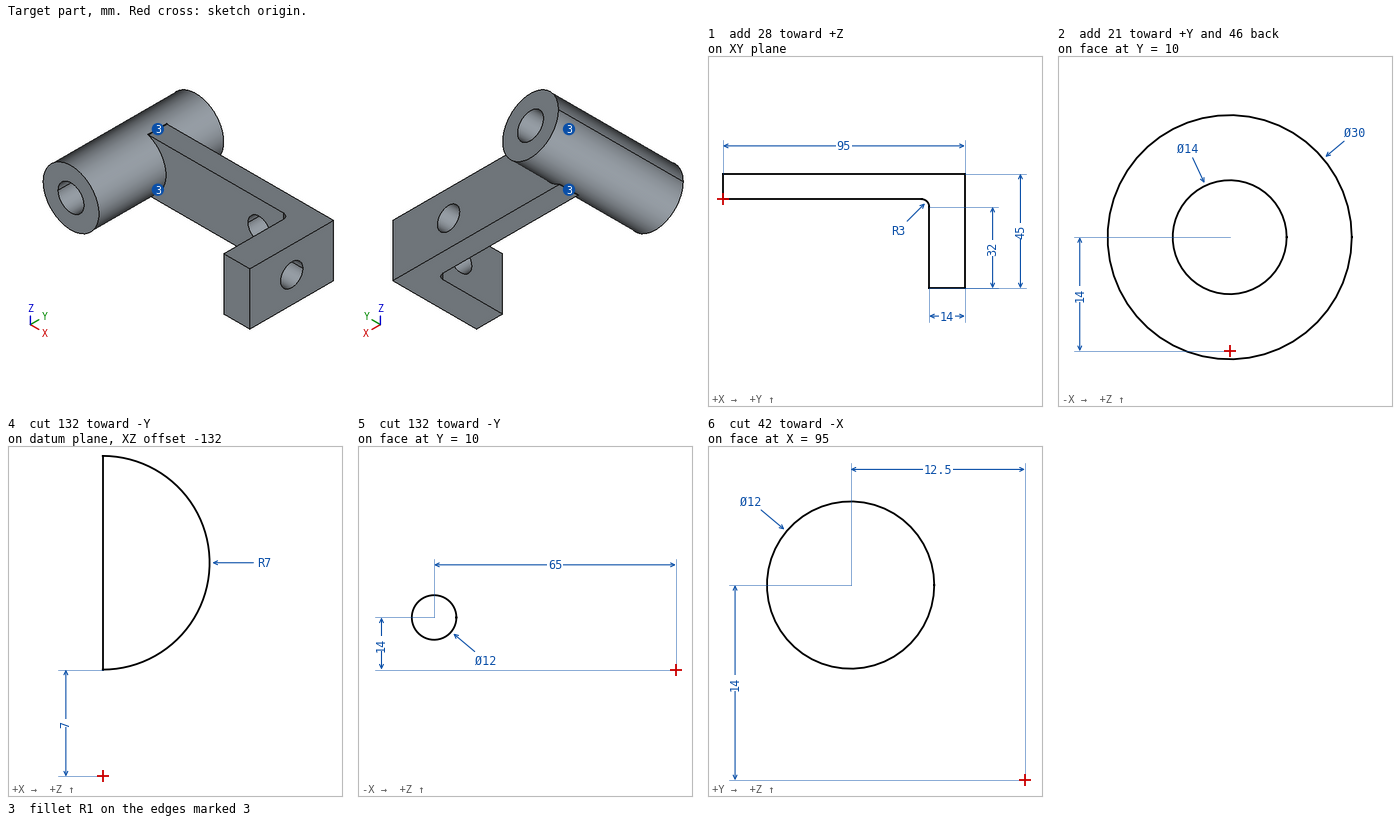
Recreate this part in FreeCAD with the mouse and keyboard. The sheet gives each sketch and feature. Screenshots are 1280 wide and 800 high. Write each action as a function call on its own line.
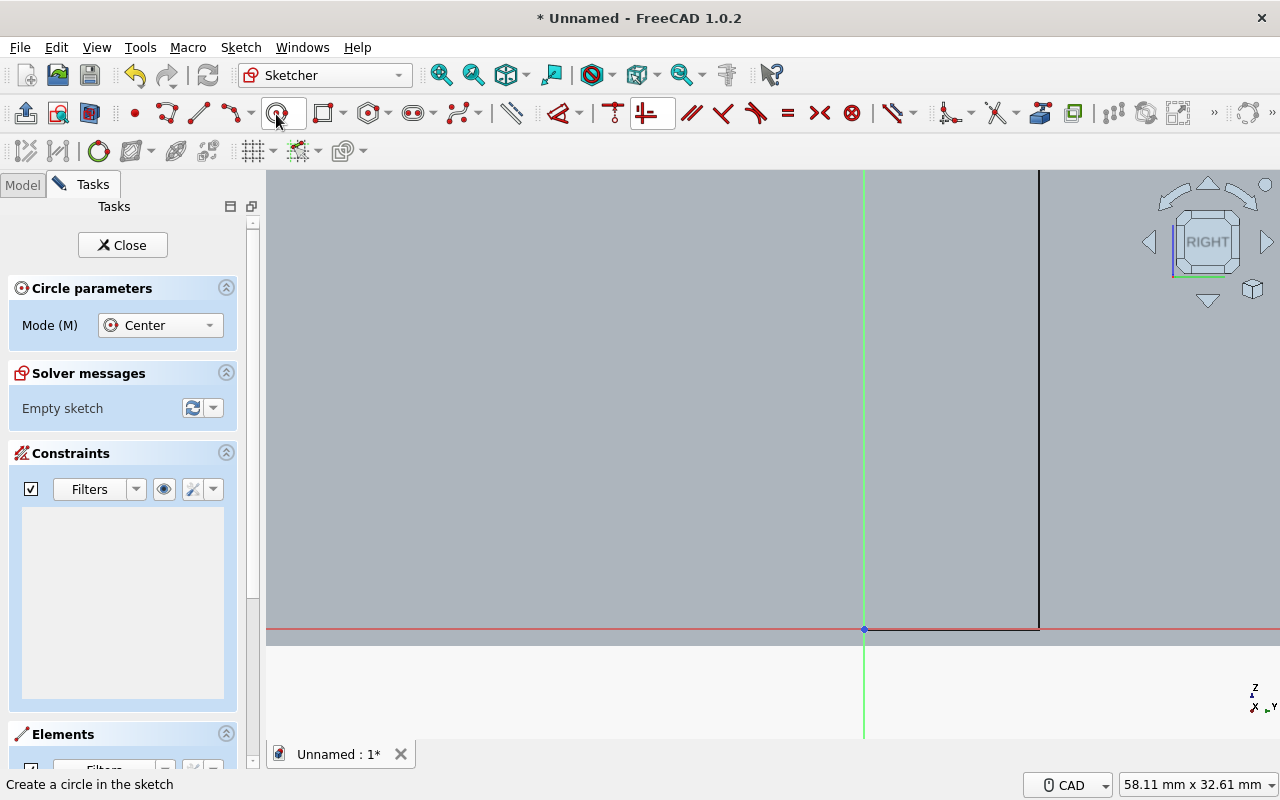
click(646, 385)
move(720, 311)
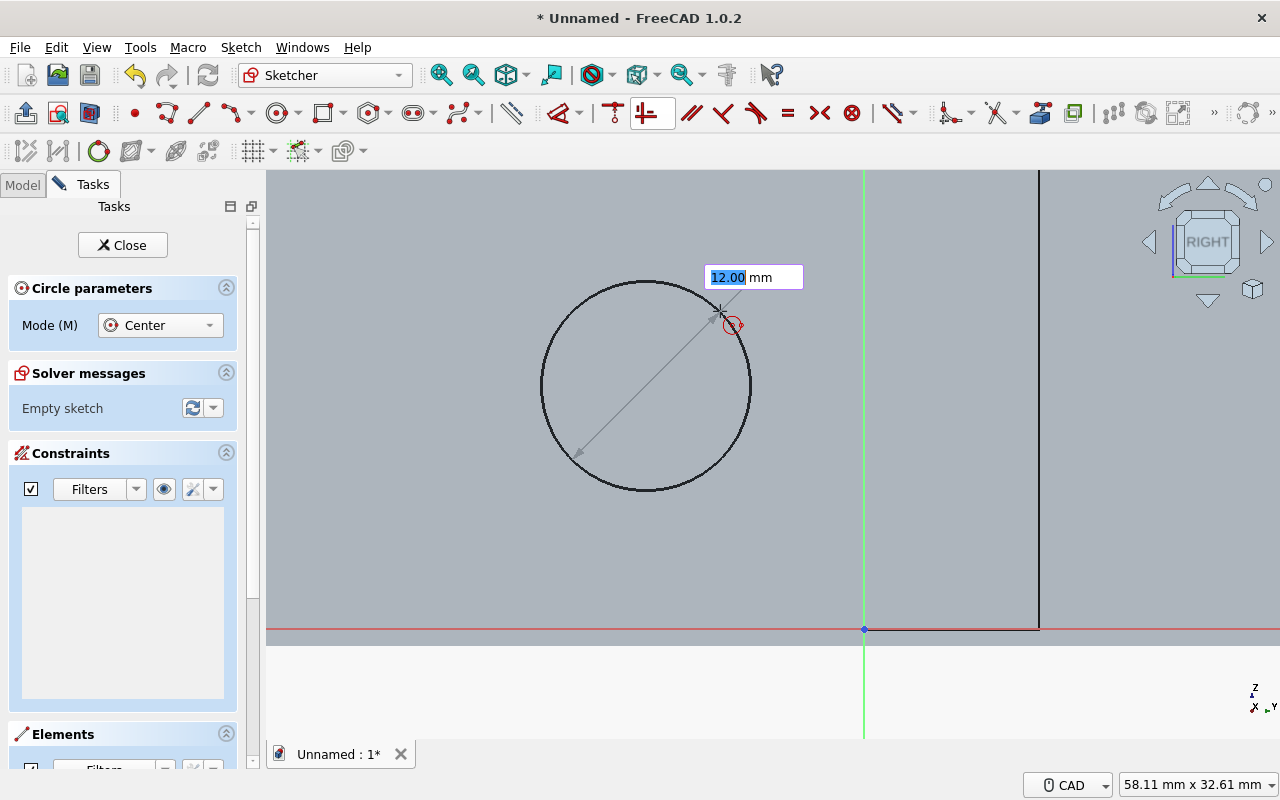
text(12)
key(Return)
key(Escape)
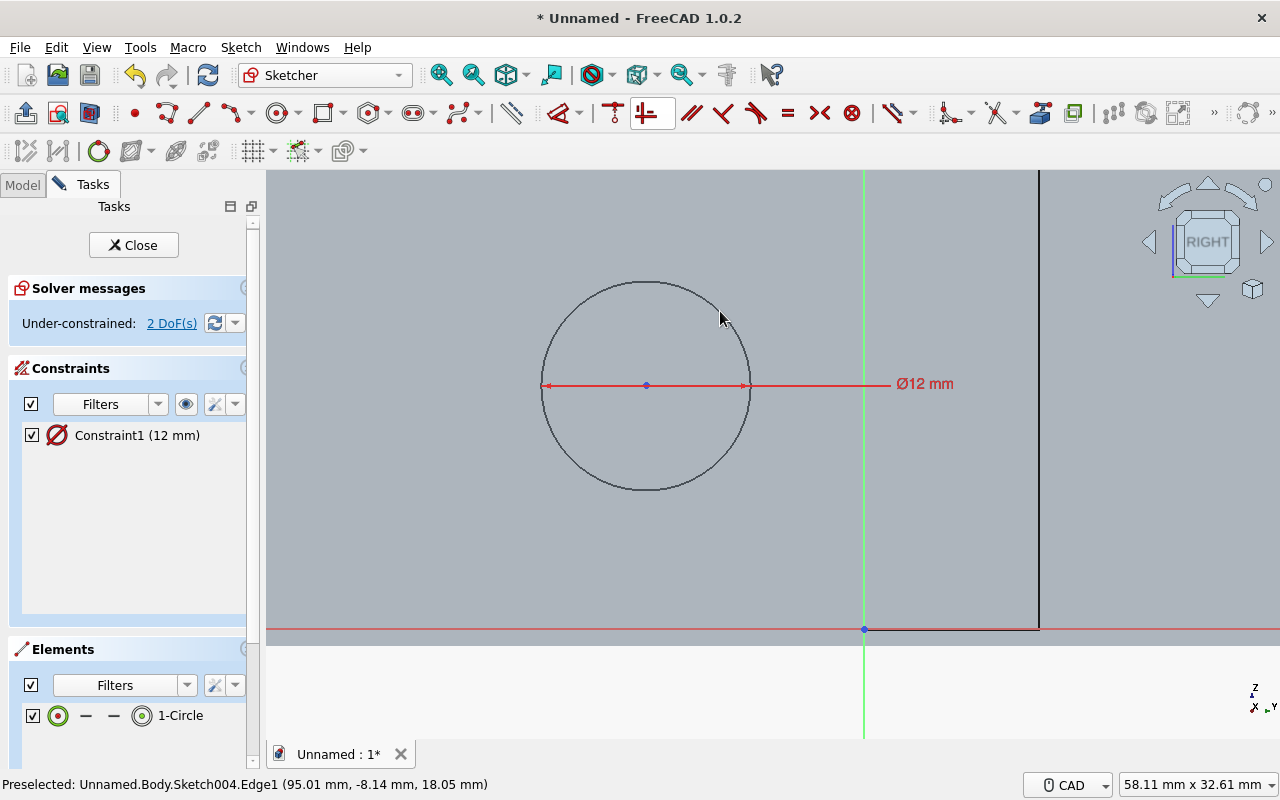
click(558, 114)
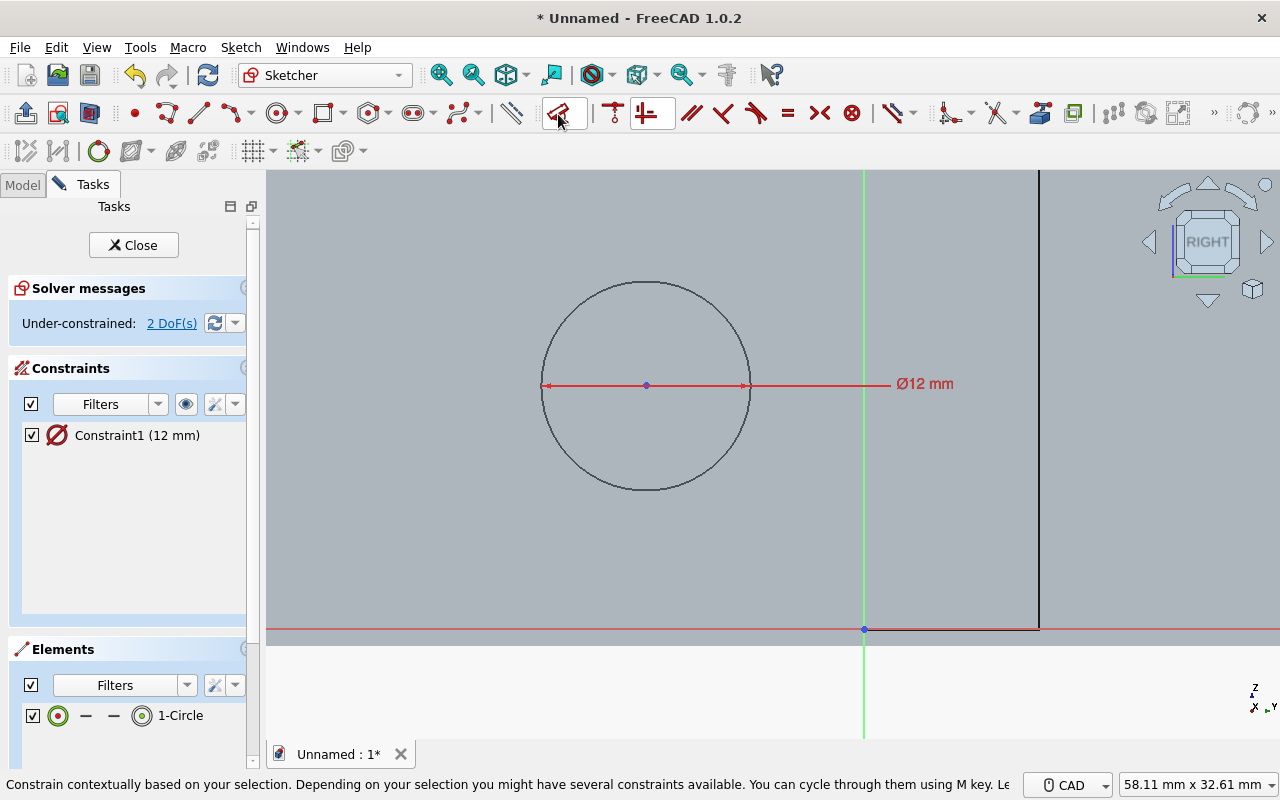
click(646, 386)
click(898, 508)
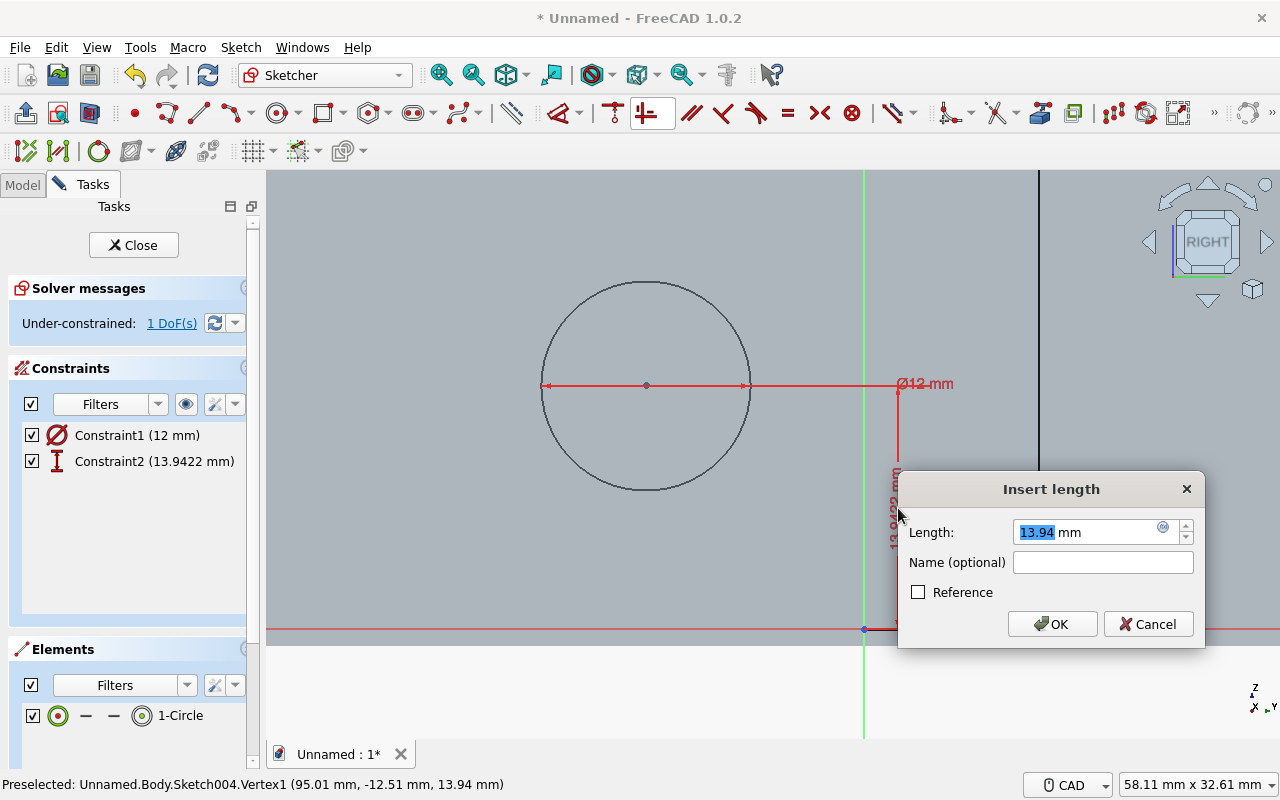
text(14)
key(Return)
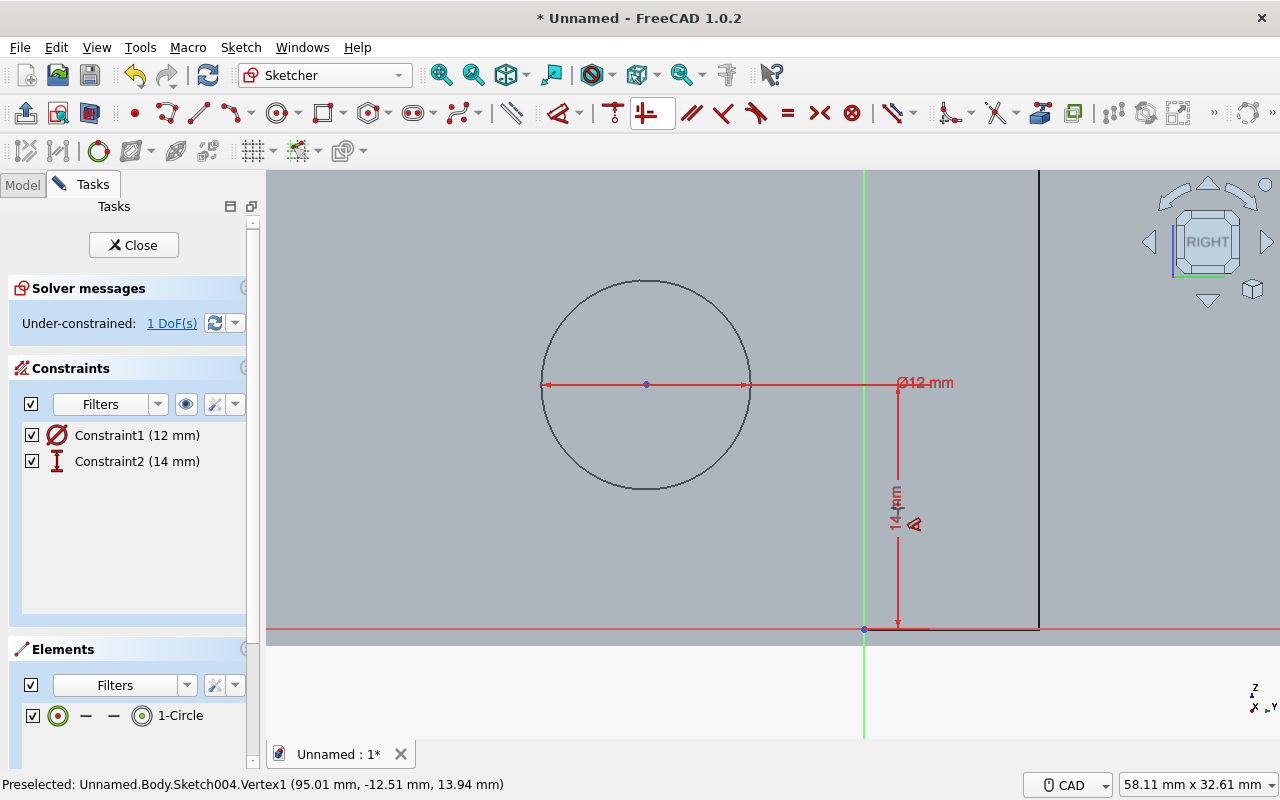
click(646, 385)
click(755, 663)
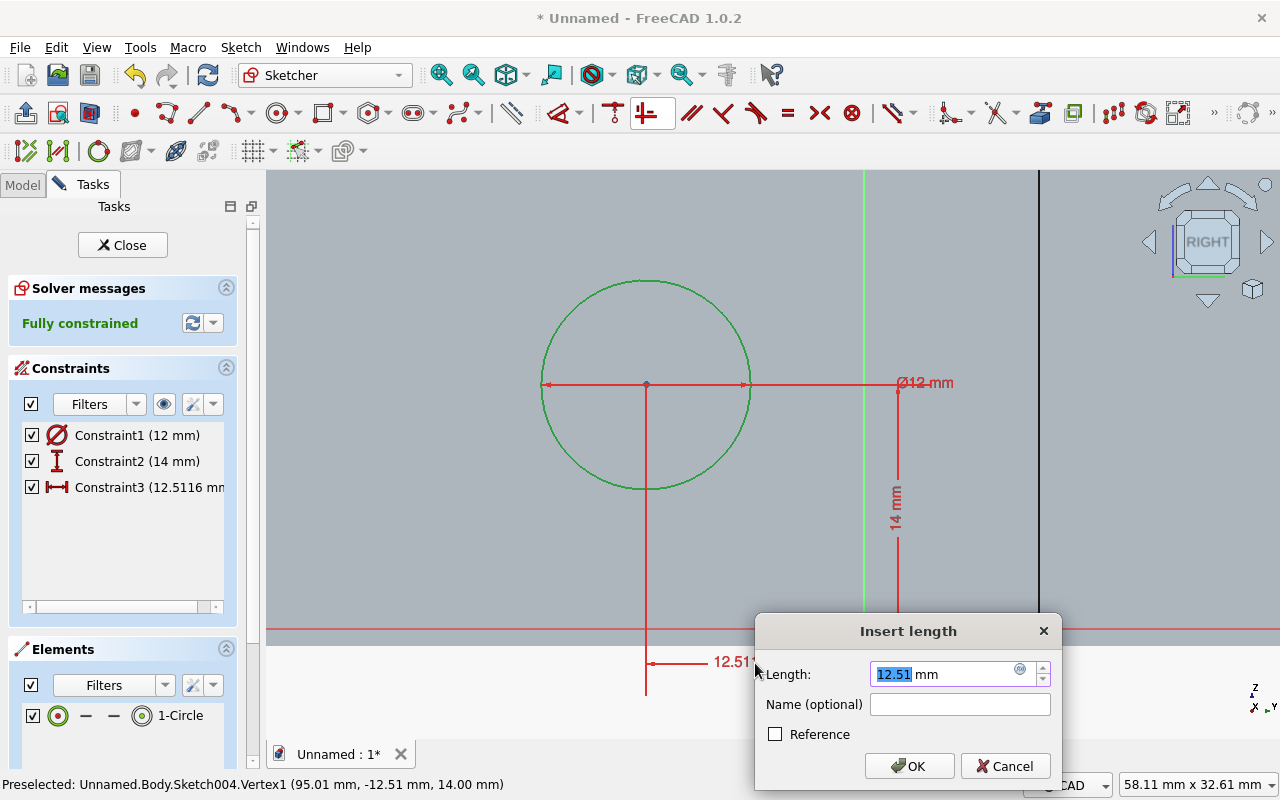
text(12.5)
key(Return)
key(Escape)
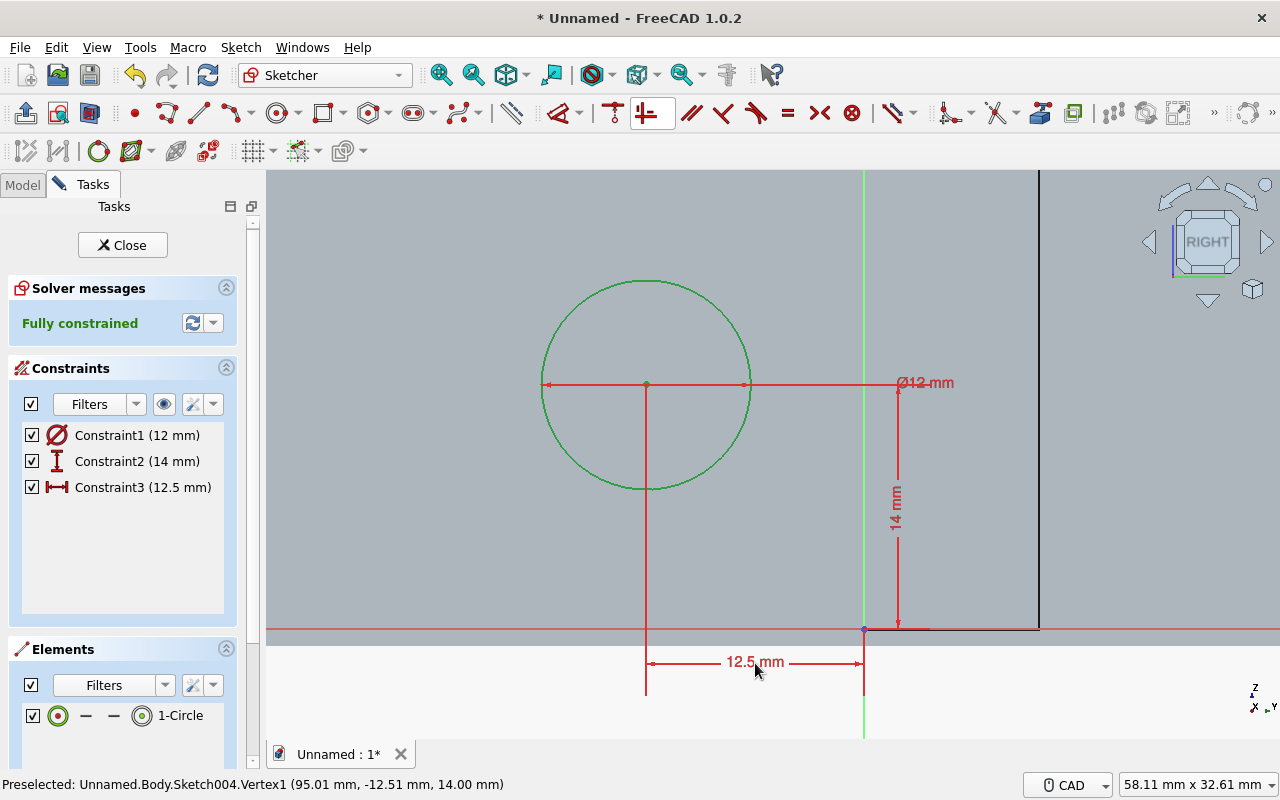
click(123, 245)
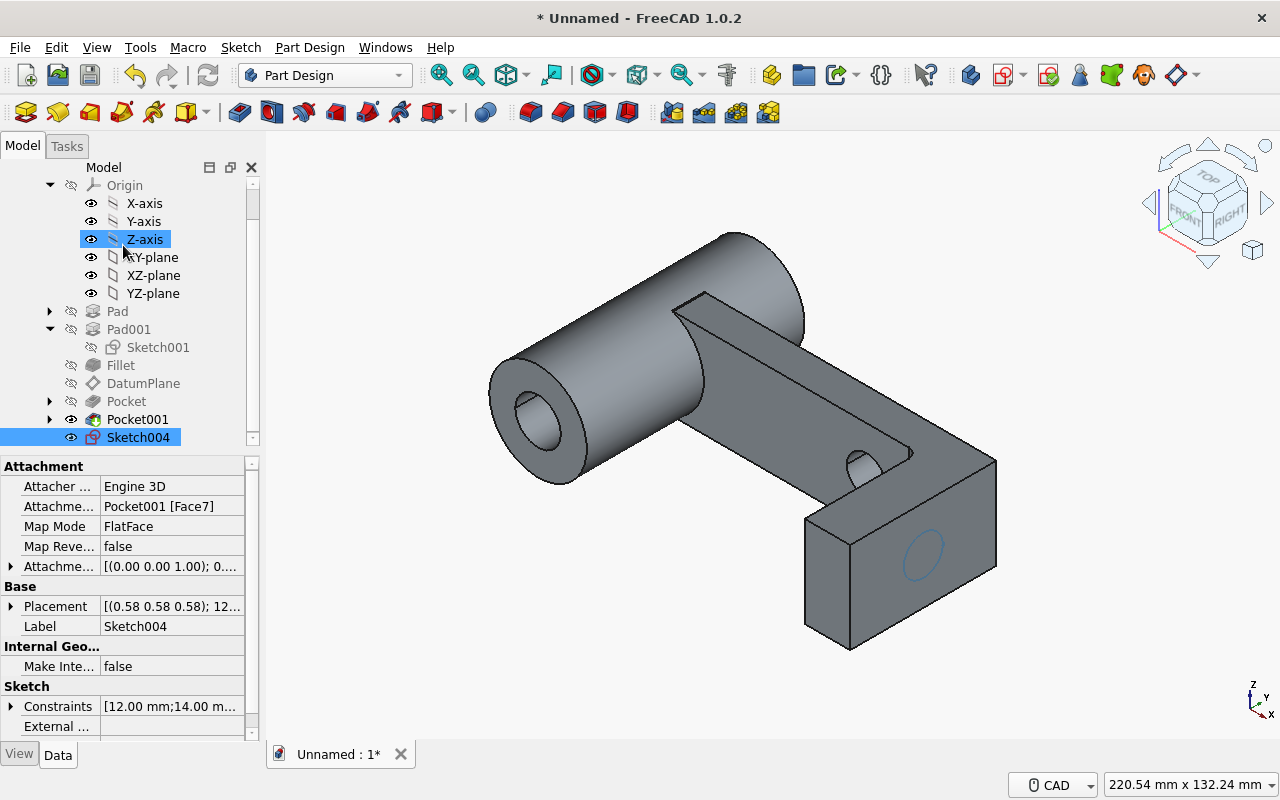
click(240, 112)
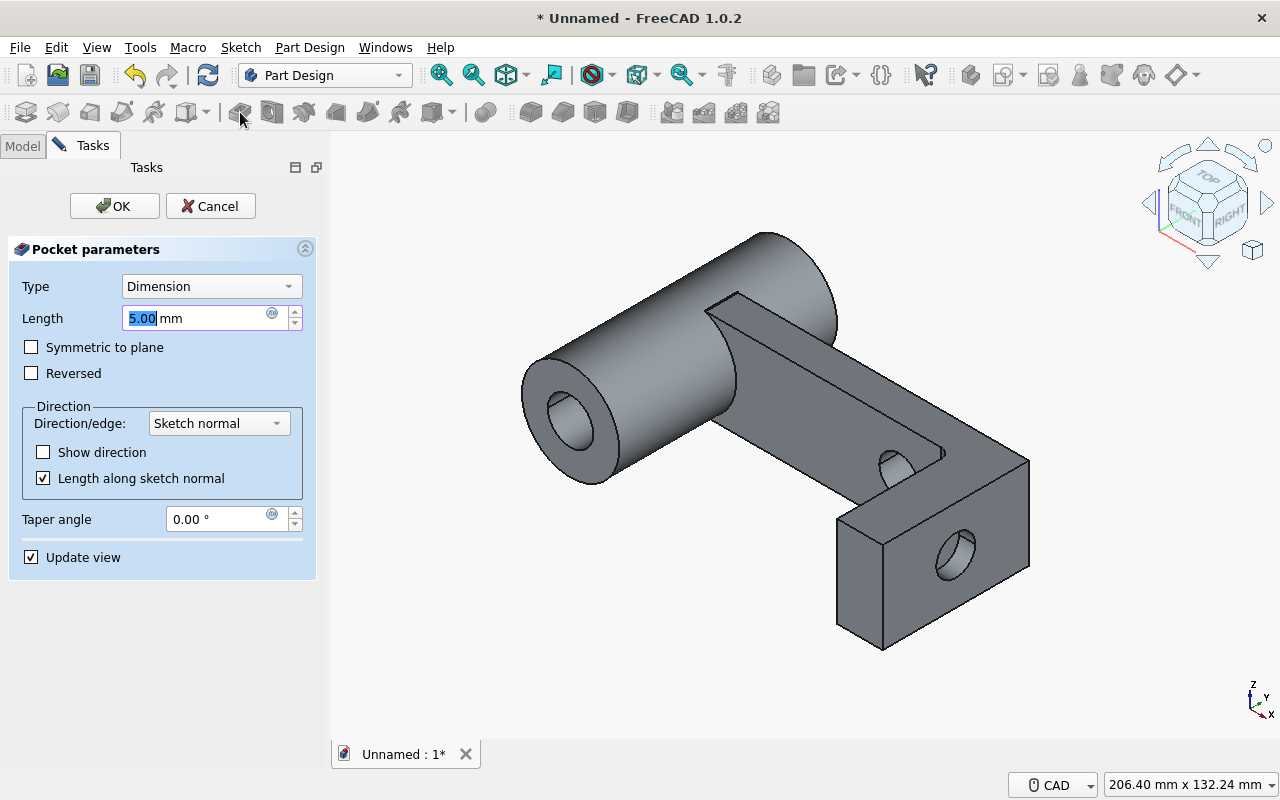
text(42)
key(Tab)